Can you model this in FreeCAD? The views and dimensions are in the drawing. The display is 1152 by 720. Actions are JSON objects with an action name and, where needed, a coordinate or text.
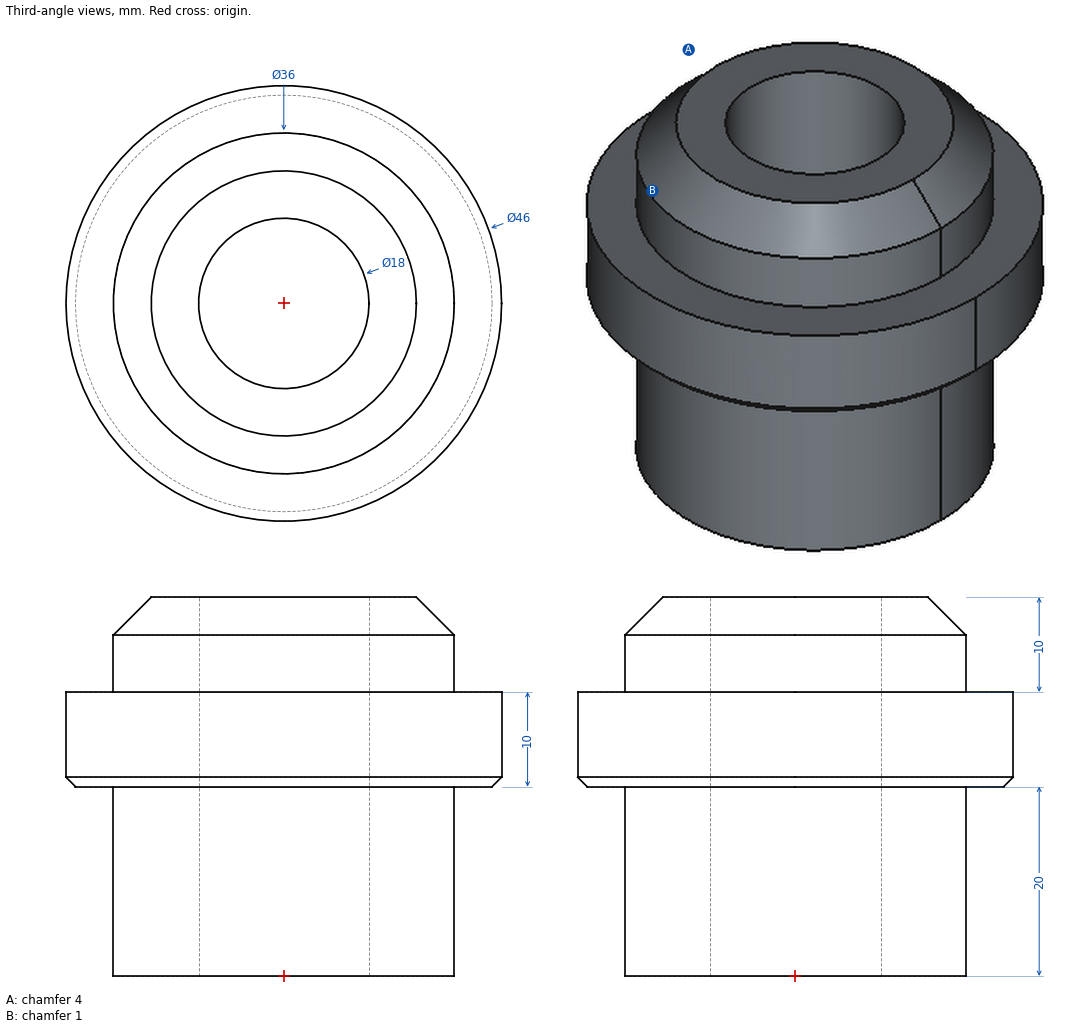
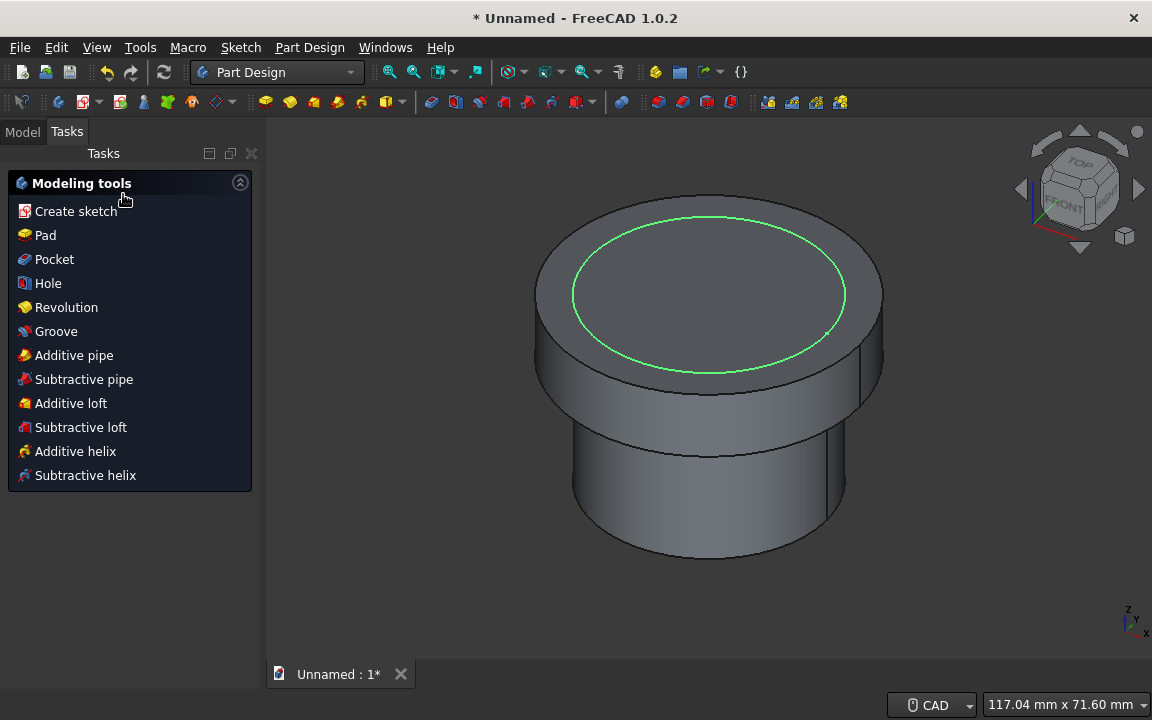
{"action": "left_click", "coordinate": [266, 102]}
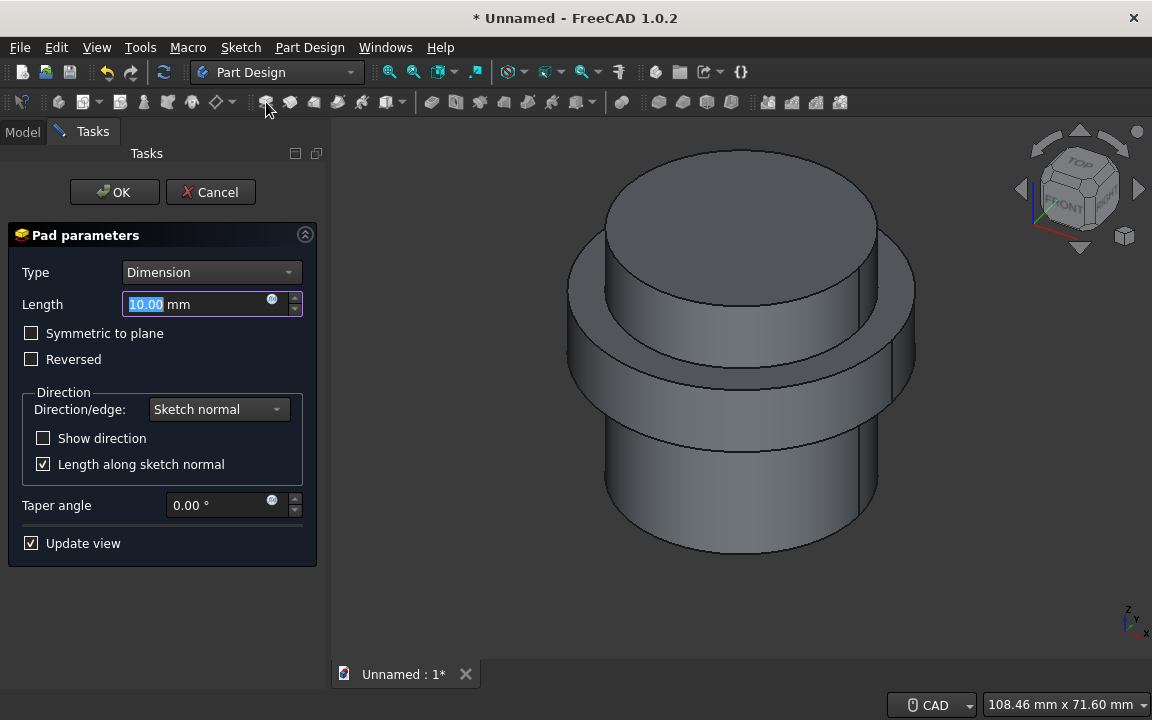
{"action": "type", "text": "10"}
{"action": "key", "text": "Tab"}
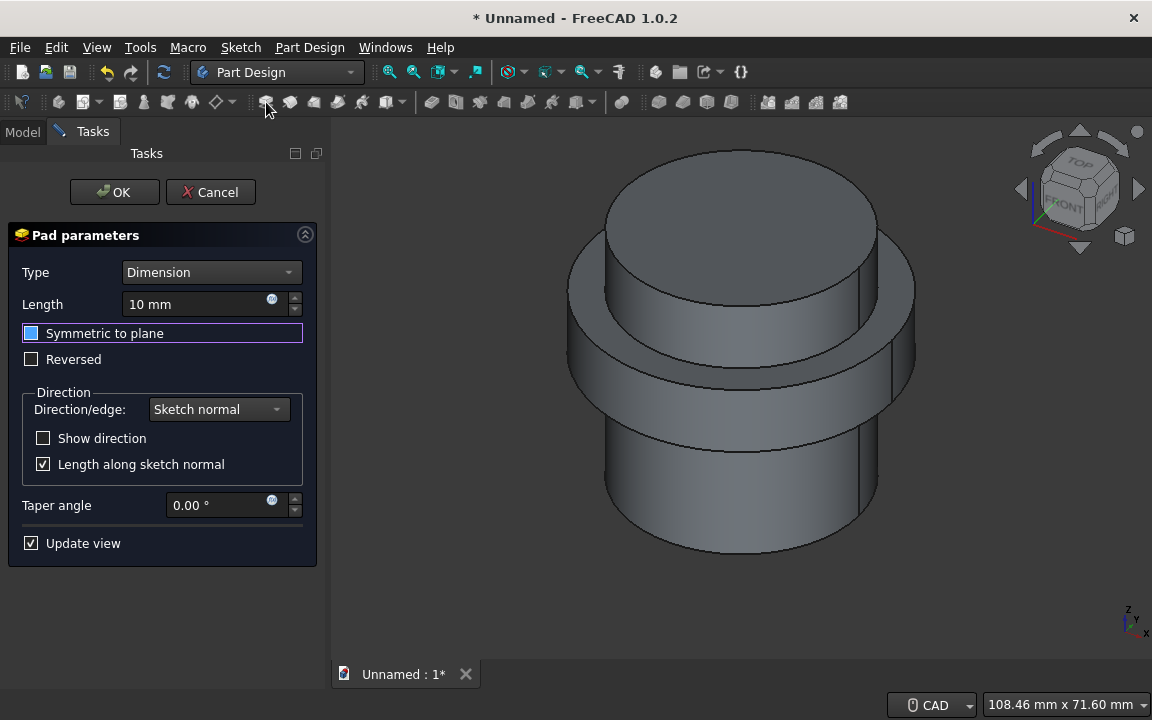
{"action": "left_click", "coordinate": [115, 192]}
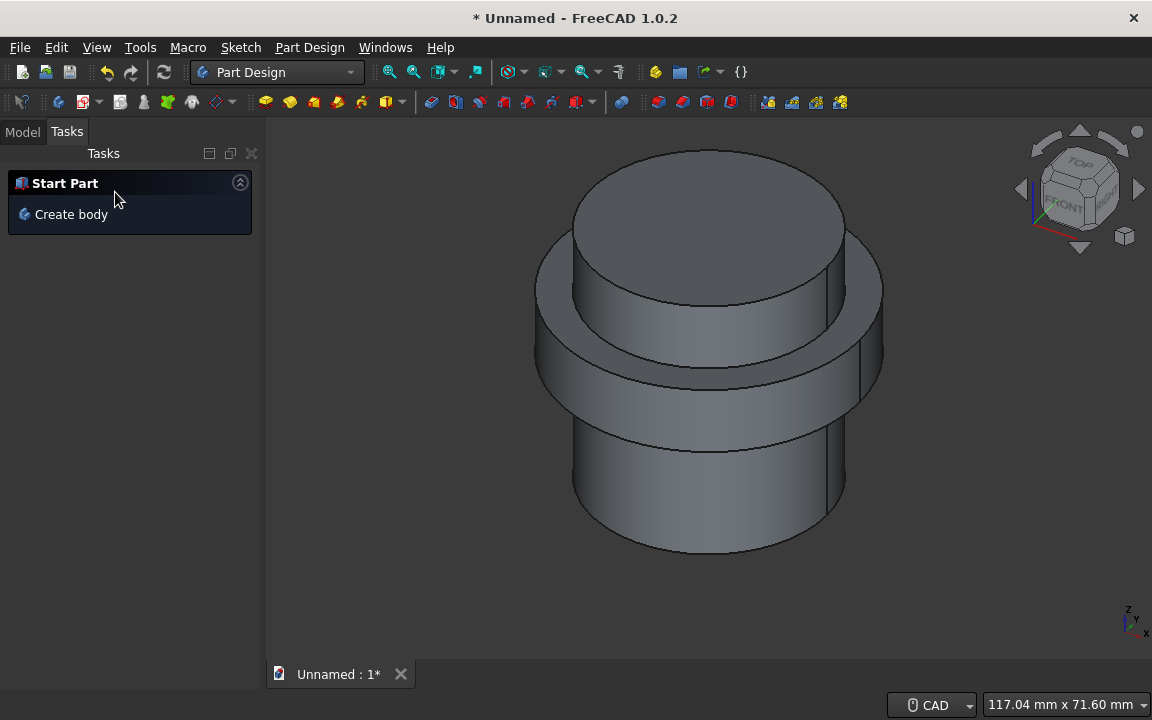
{"action": "left_click", "coordinate": [390, 72]}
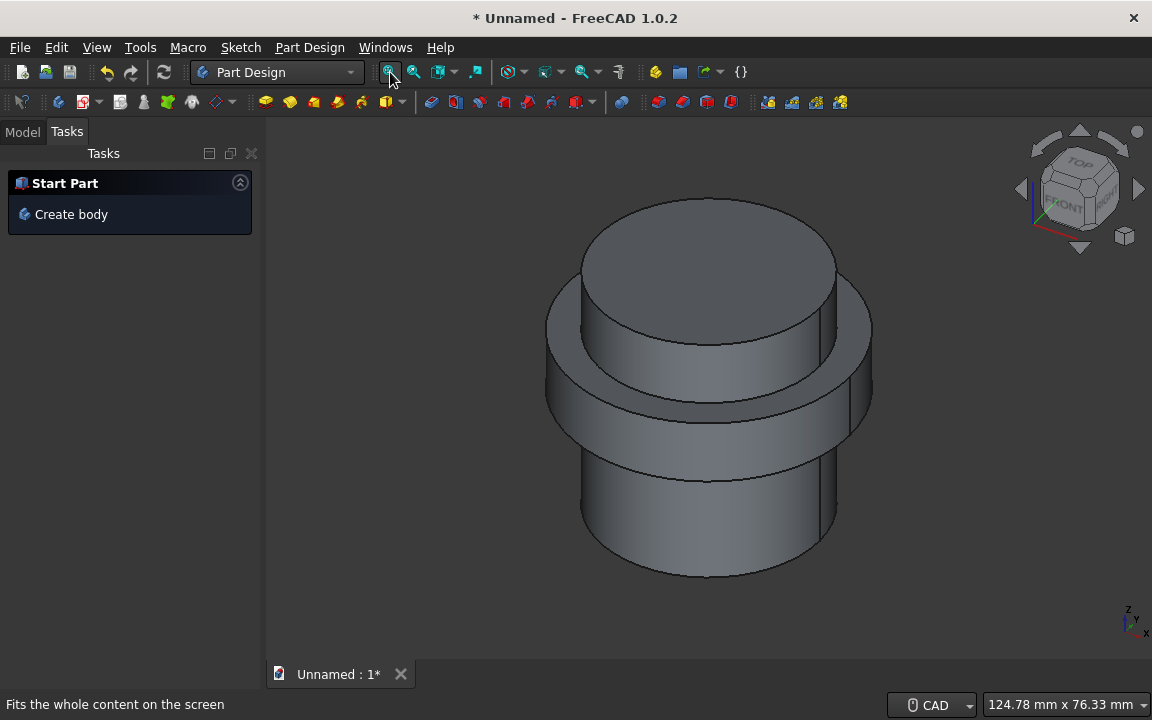
{"action": "left_click", "coordinate": [582, 278]}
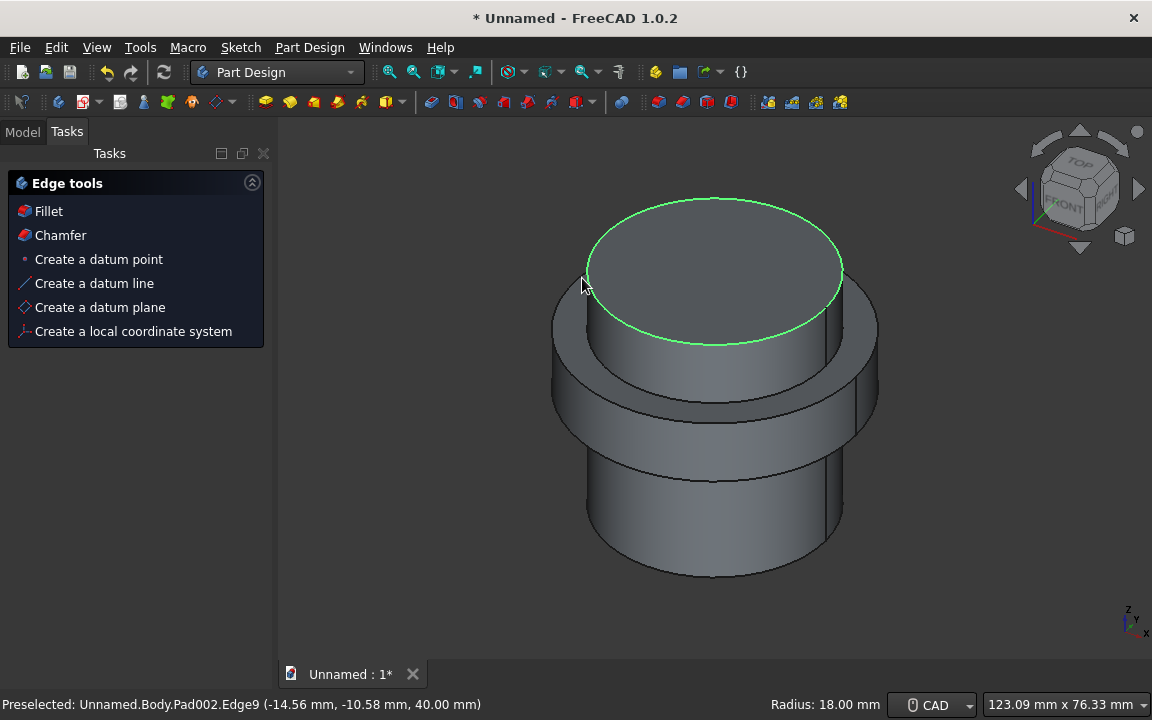
{"action": "left_click", "coordinate": [684, 102]}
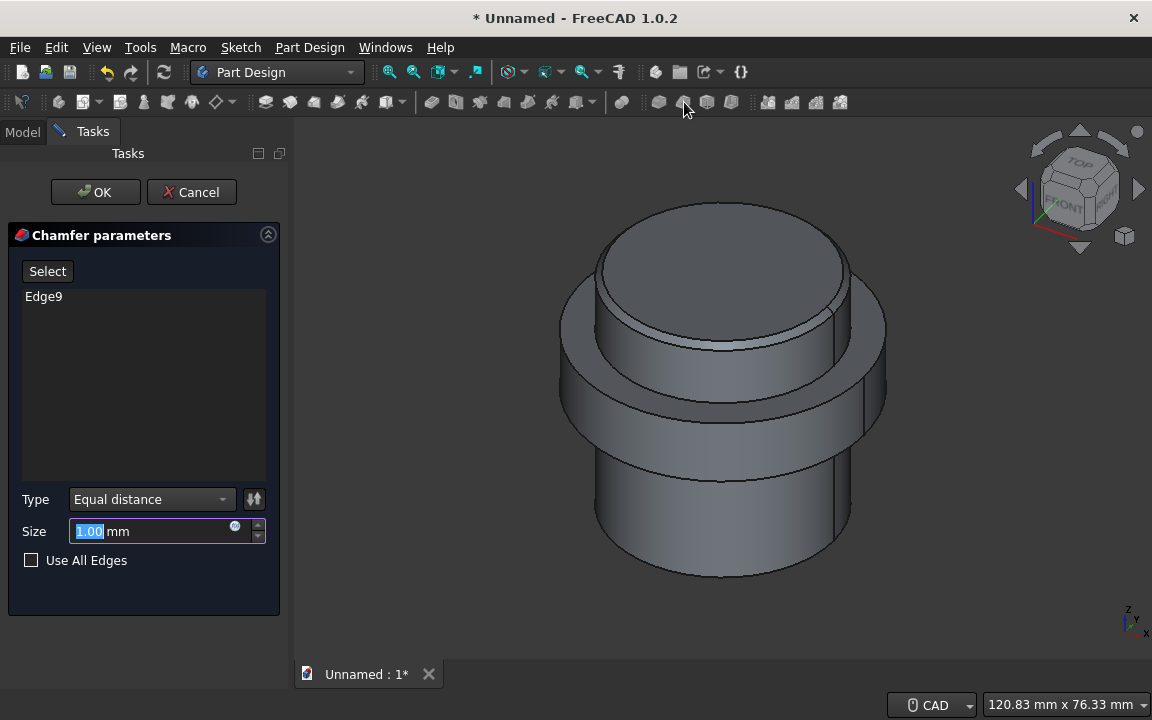
{"action": "type", "text": "4"}
{"action": "key", "text": "Tab"}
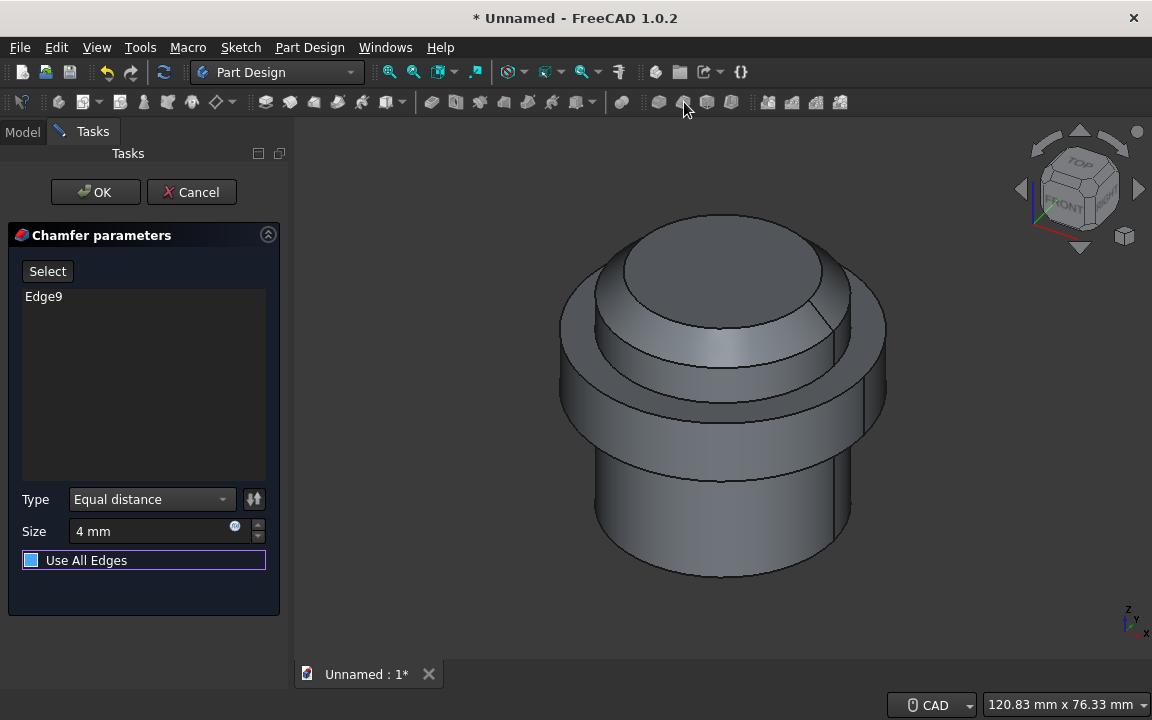
{"action": "left_click", "coordinate": [96, 192]}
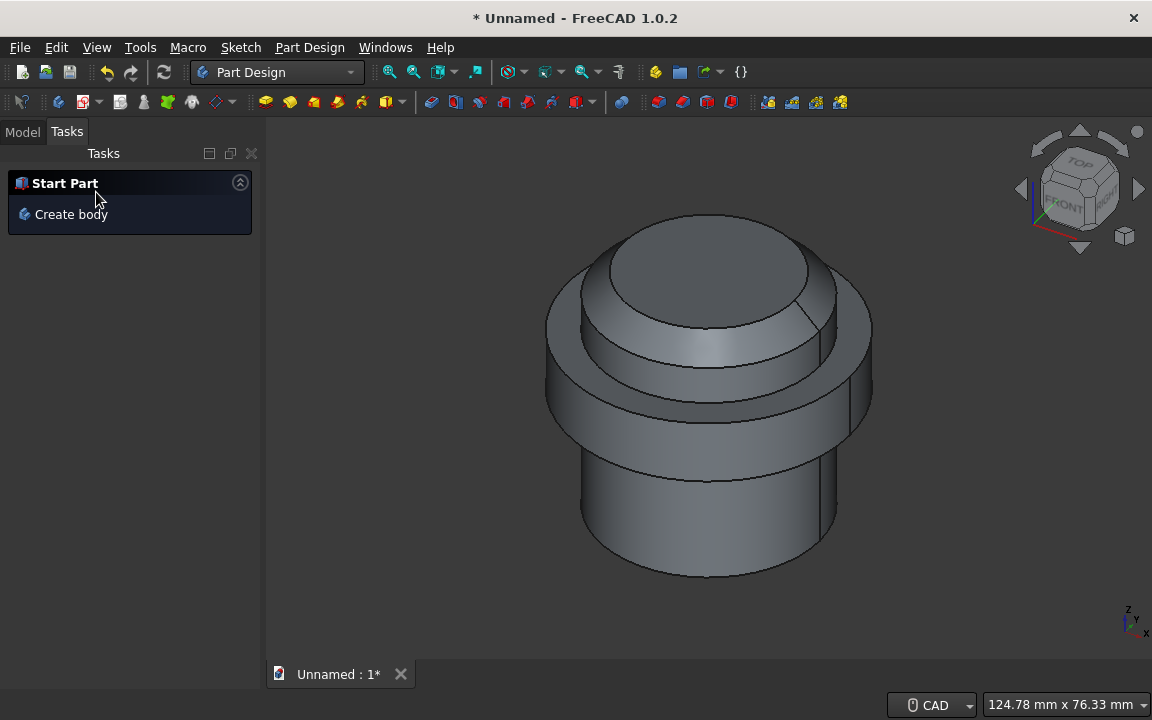
{"action": "left_click", "coordinate": [709, 271]}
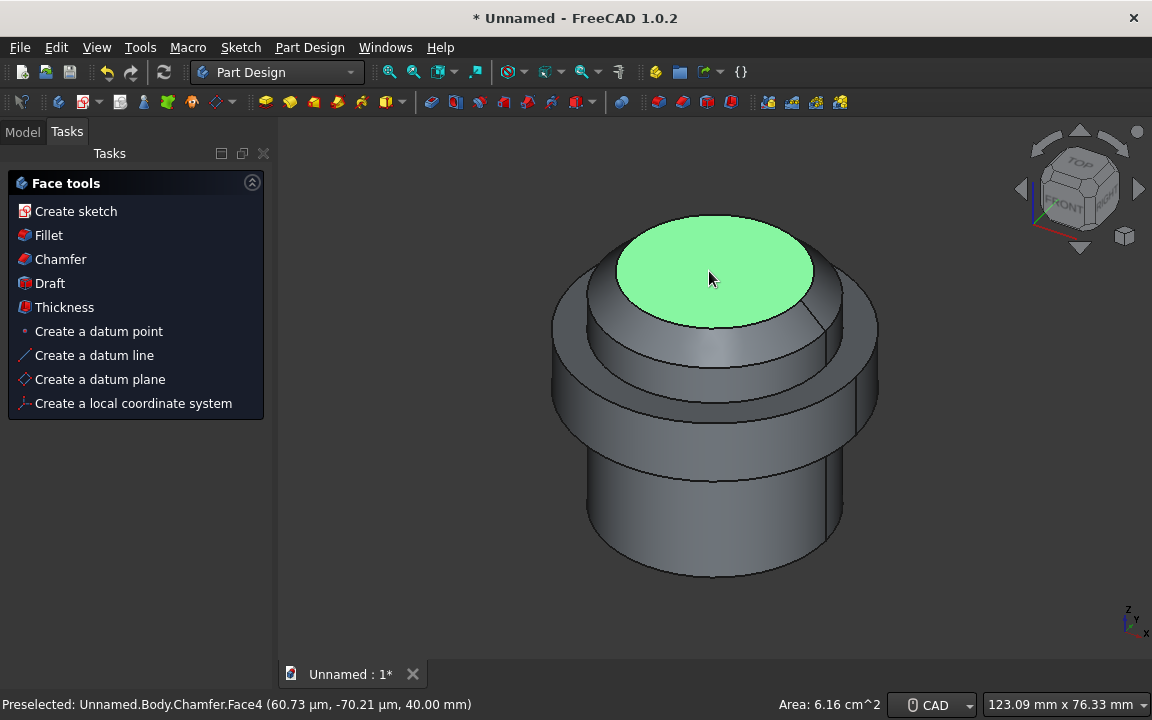
{"action": "left_click", "coordinate": [84, 102]}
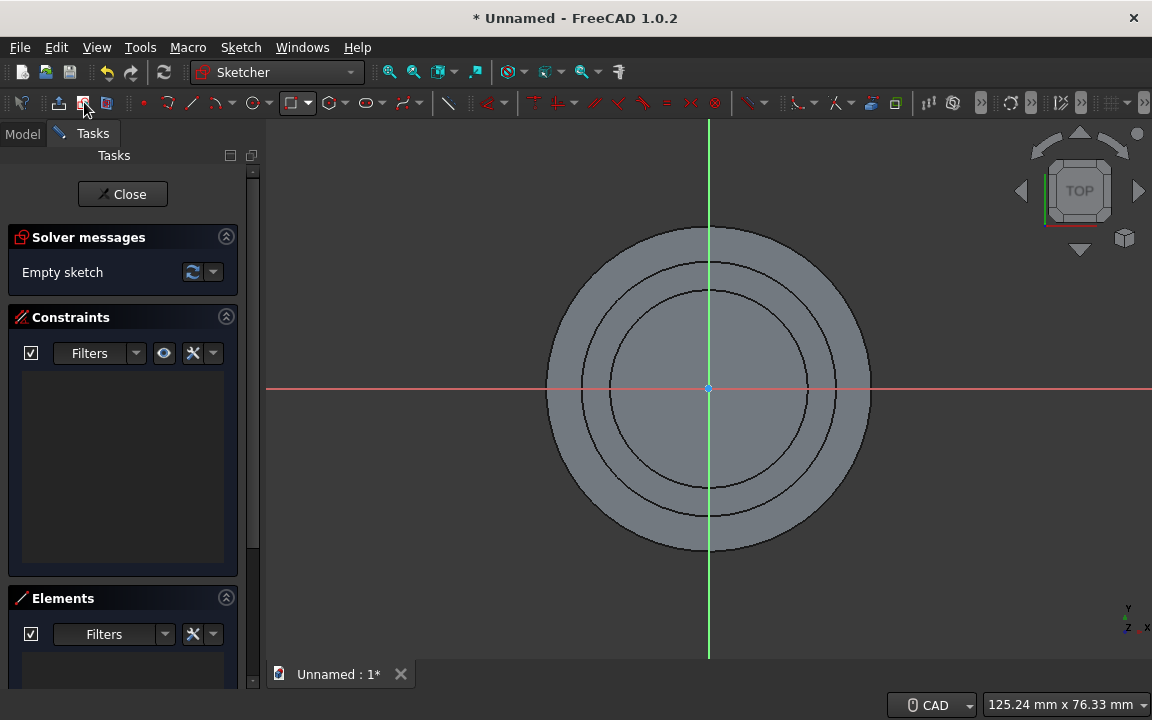
{"action": "scroll", "coordinate": [749, 389], "scroll_direction": "up", "scroll_amount": 5}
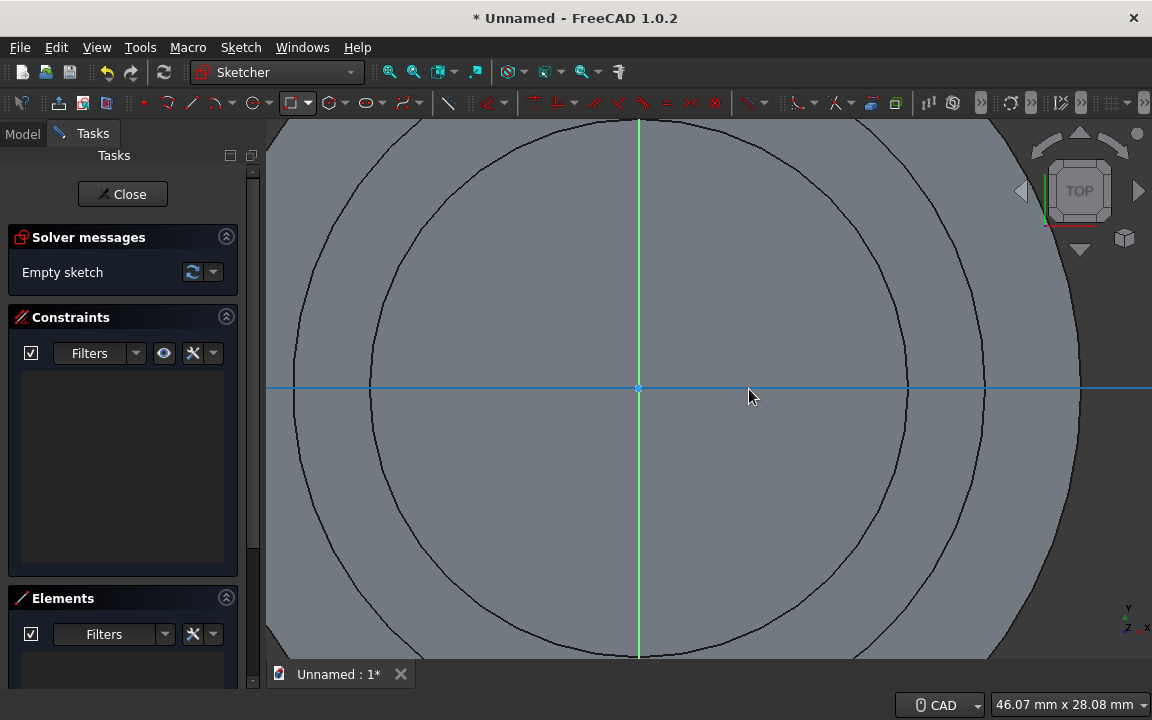
{"action": "key", "text": "g c"}